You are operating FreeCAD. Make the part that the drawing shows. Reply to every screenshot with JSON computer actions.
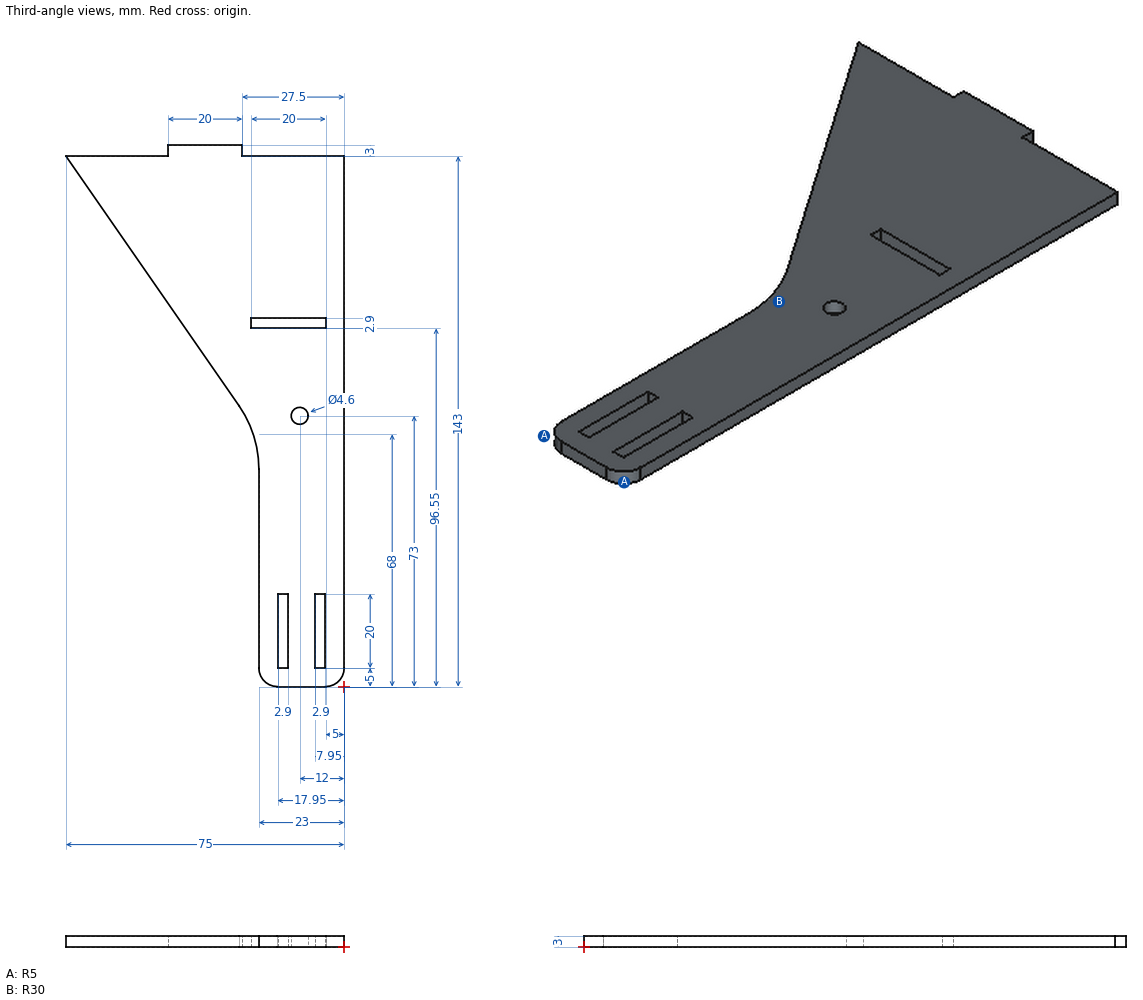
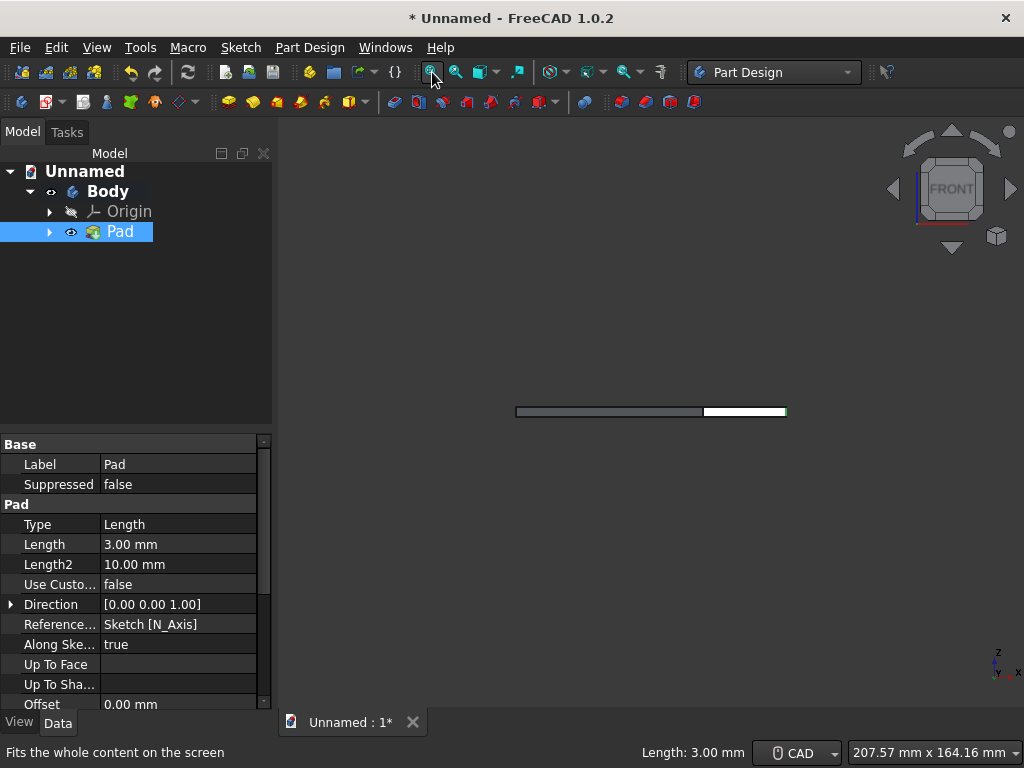
{"action": "left_click", "coordinate": [432, 72]}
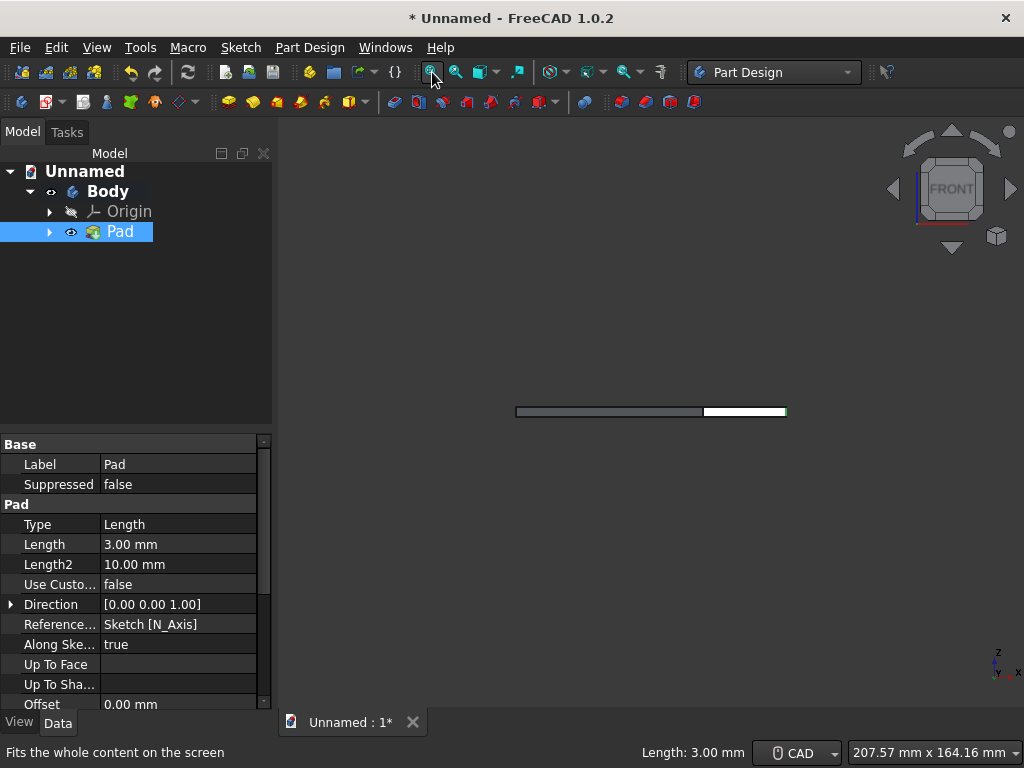
{"action": "scroll", "coordinate": [703, 411], "scroll_direction": "up", "scroll_amount": 7}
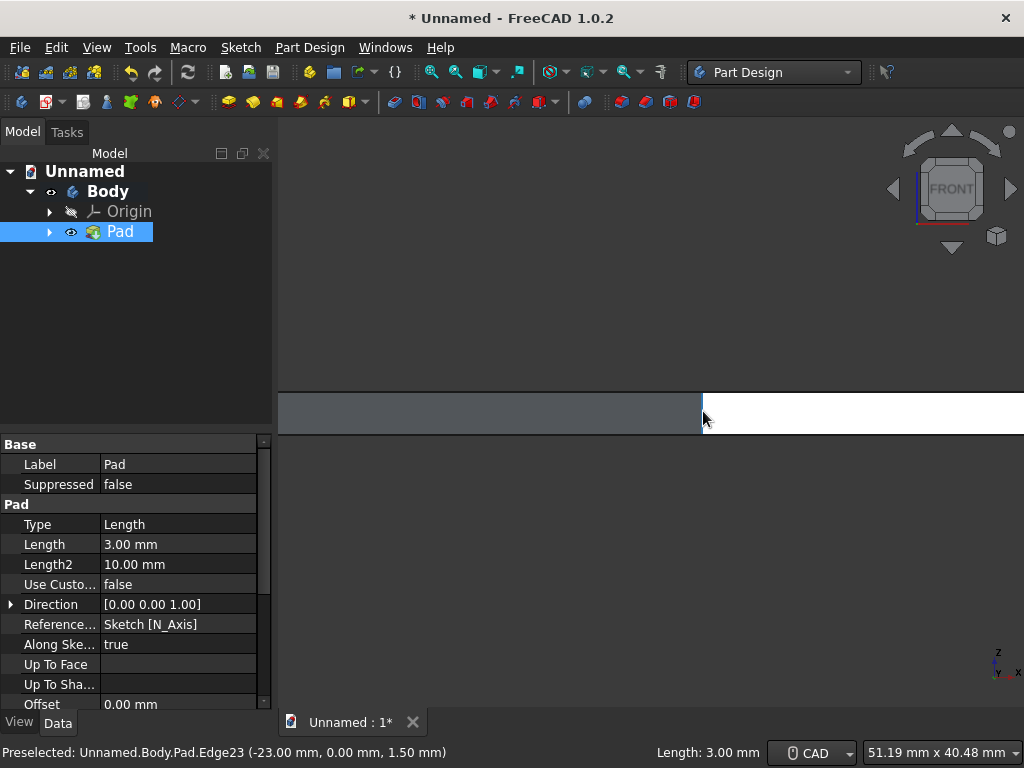
{"action": "left_click", "coordinate": [702, 413], "text": "ctrl"}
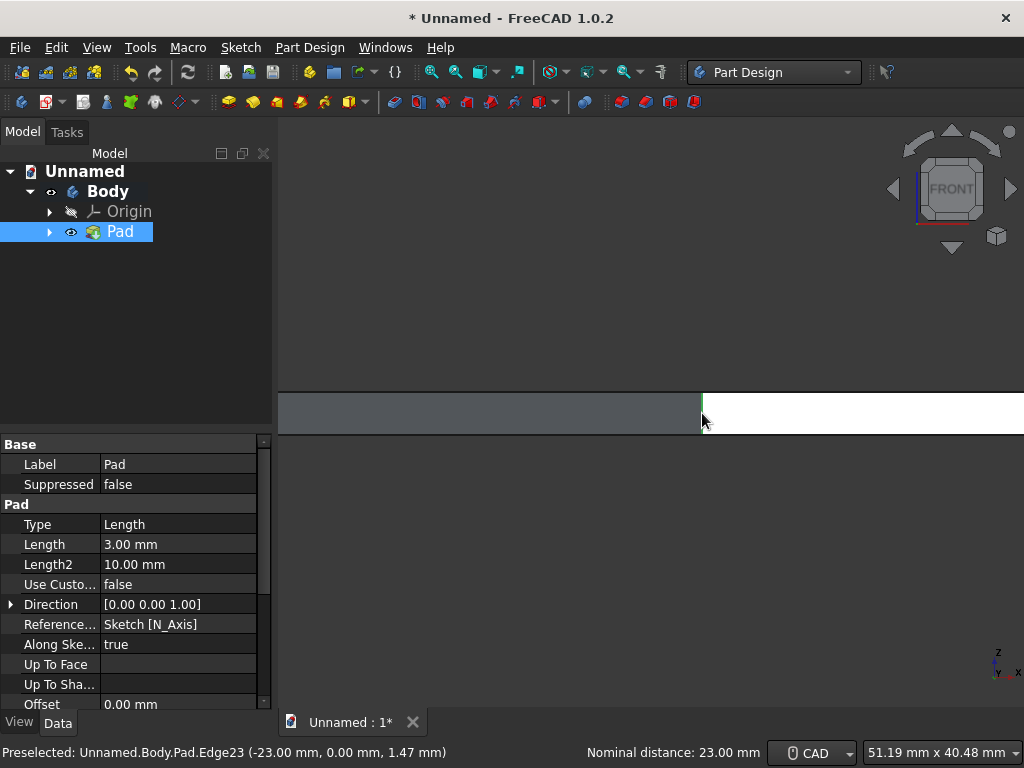
{"action": "left_click", "coordinate": [622, 102]}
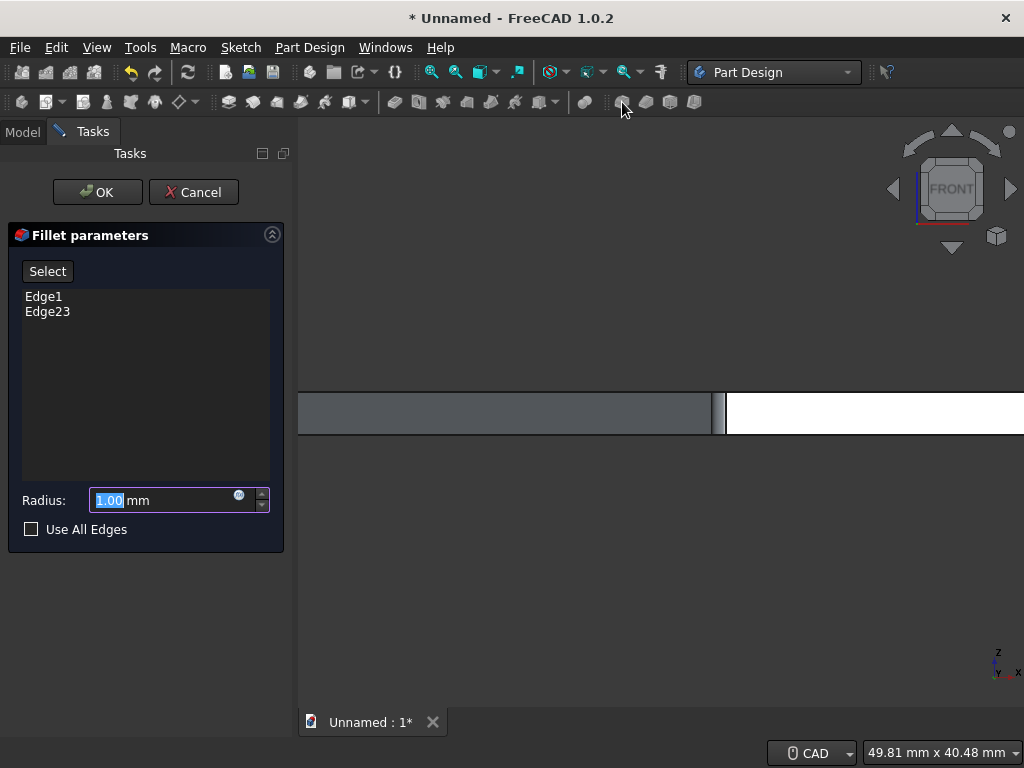
{"action": "type", "text": "5"}
{"action": "key", "text": "Tab"}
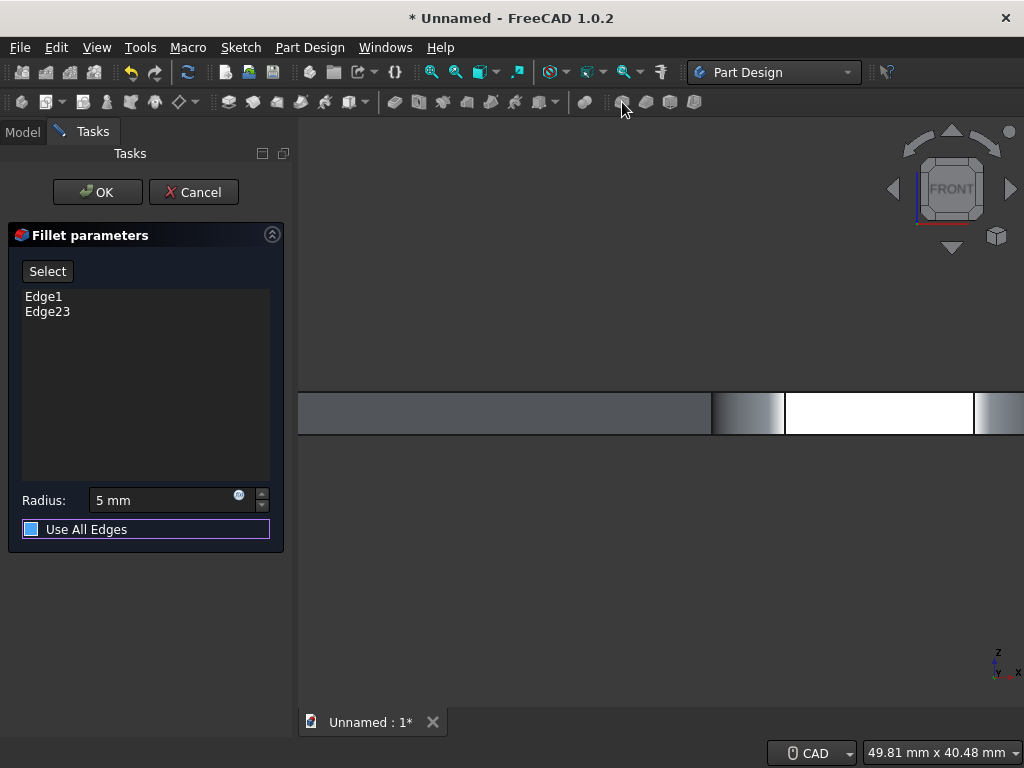
{"action": "left_click", "coordinate": [98, 192]}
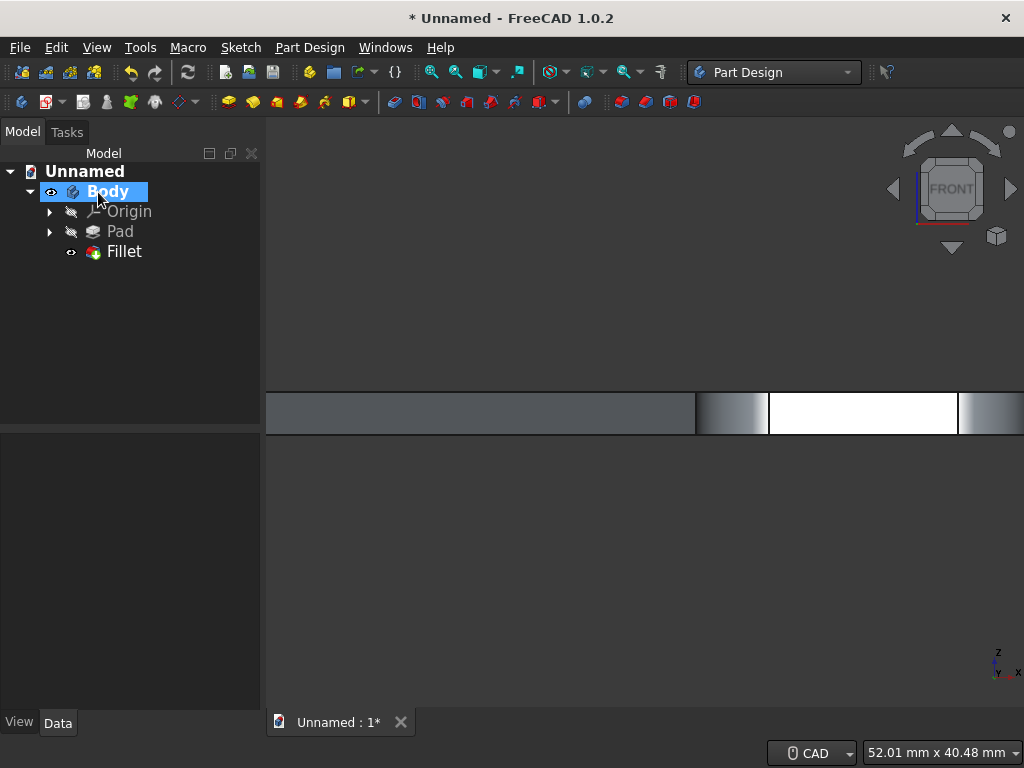
{"action": "key", "text": "v f"}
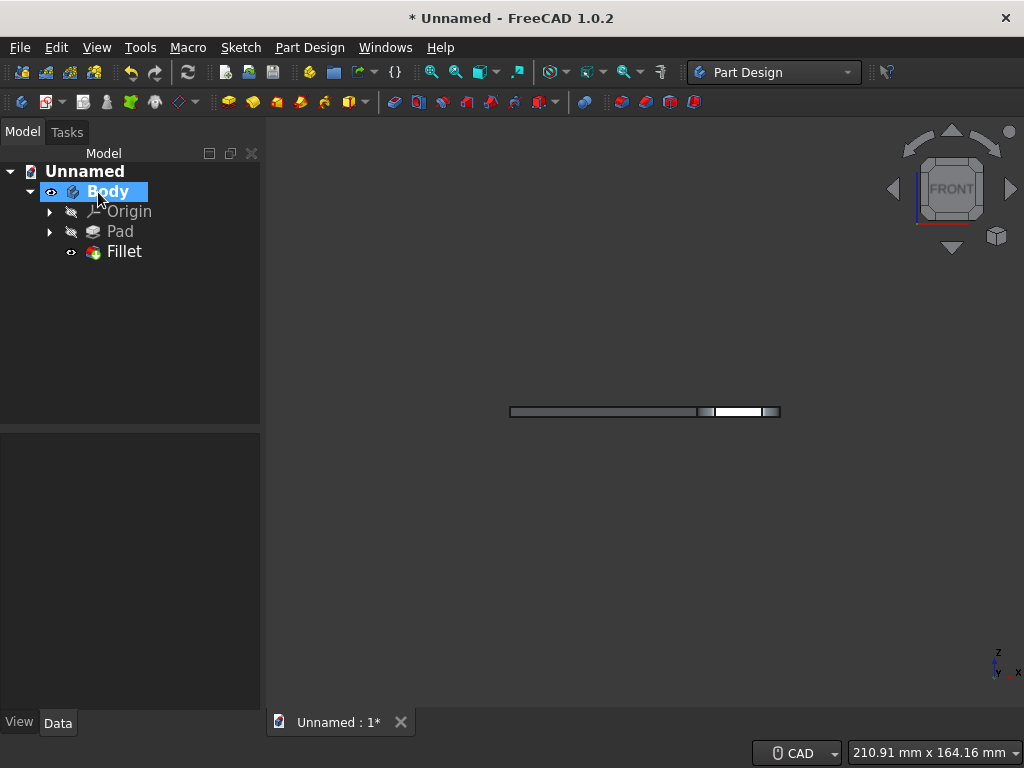
{"action": "scroll", "coordinate": [697, 411], "scroll_direction": "up", "scroll_amount": 7}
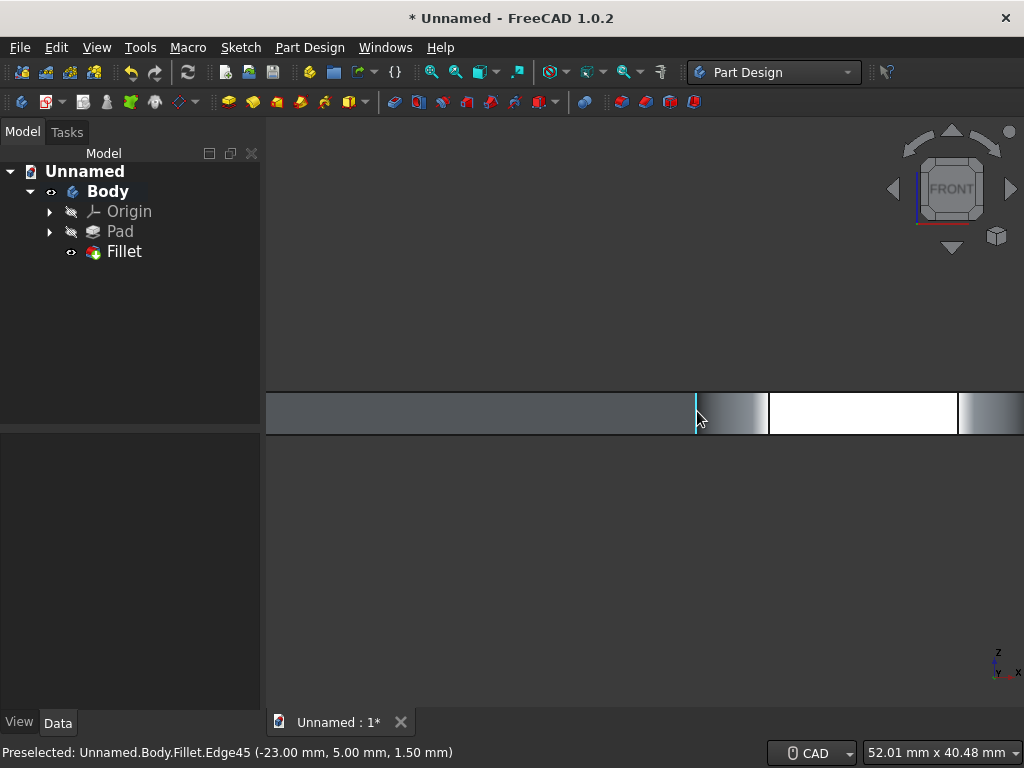
{"action": "key", "text": "v f"}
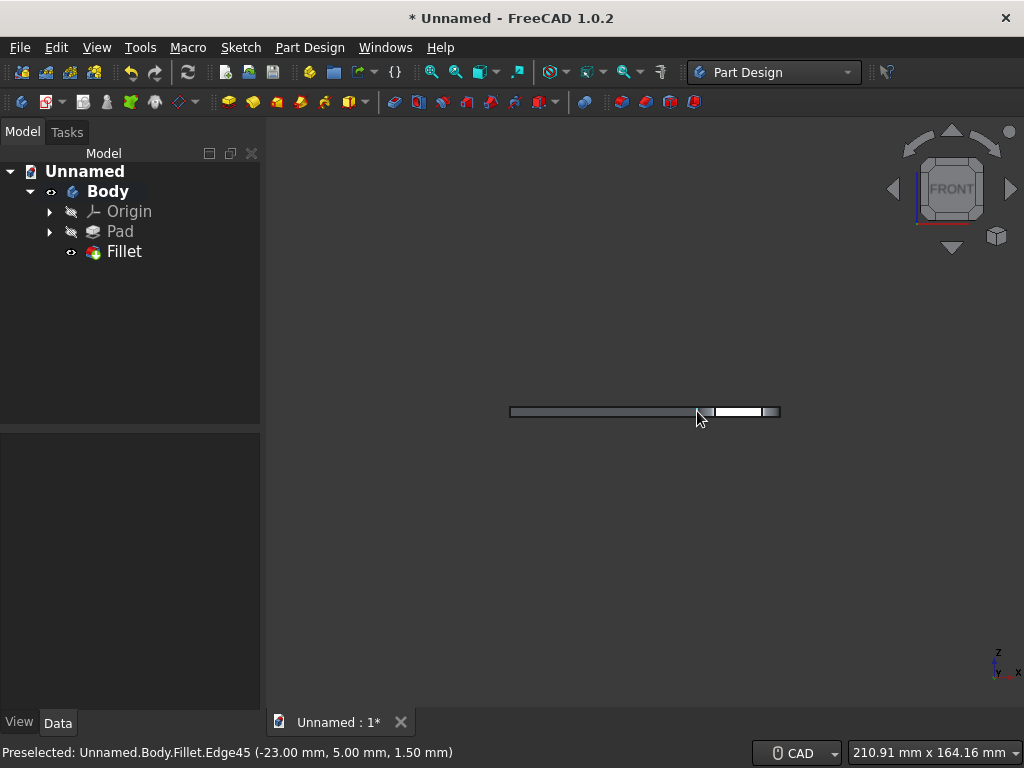
{"action": "key", "text": "0"}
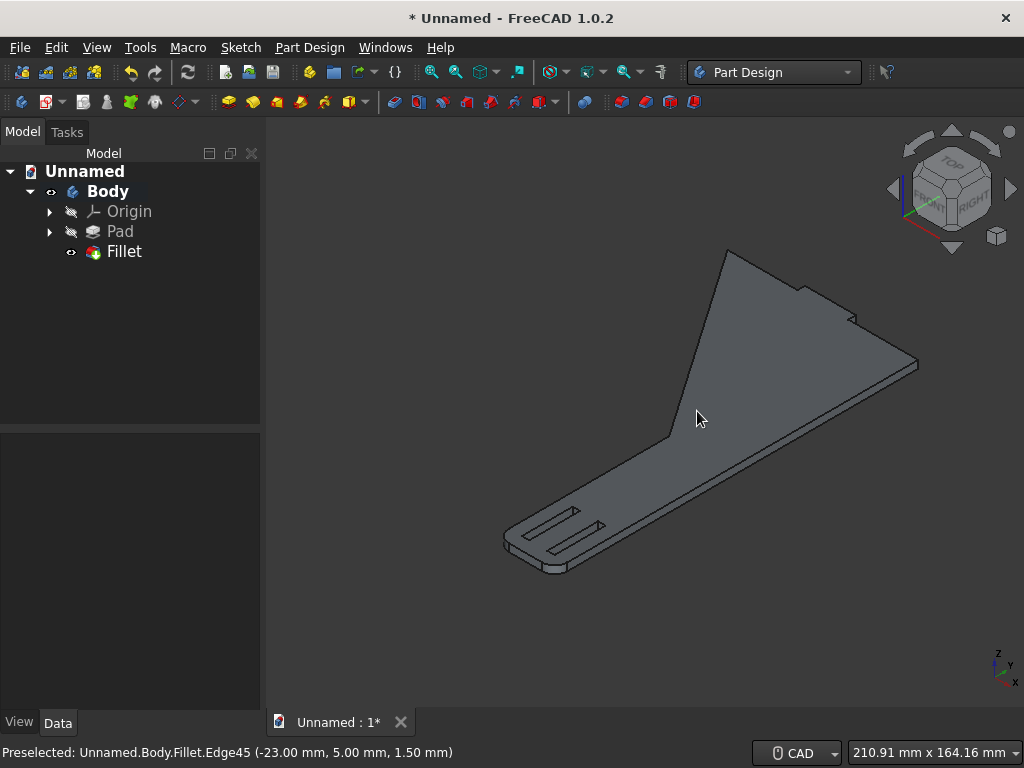
{"action": "scroll", "coordinate": [669, 440], "scroll_direction": "up", "scroll_amount": 7}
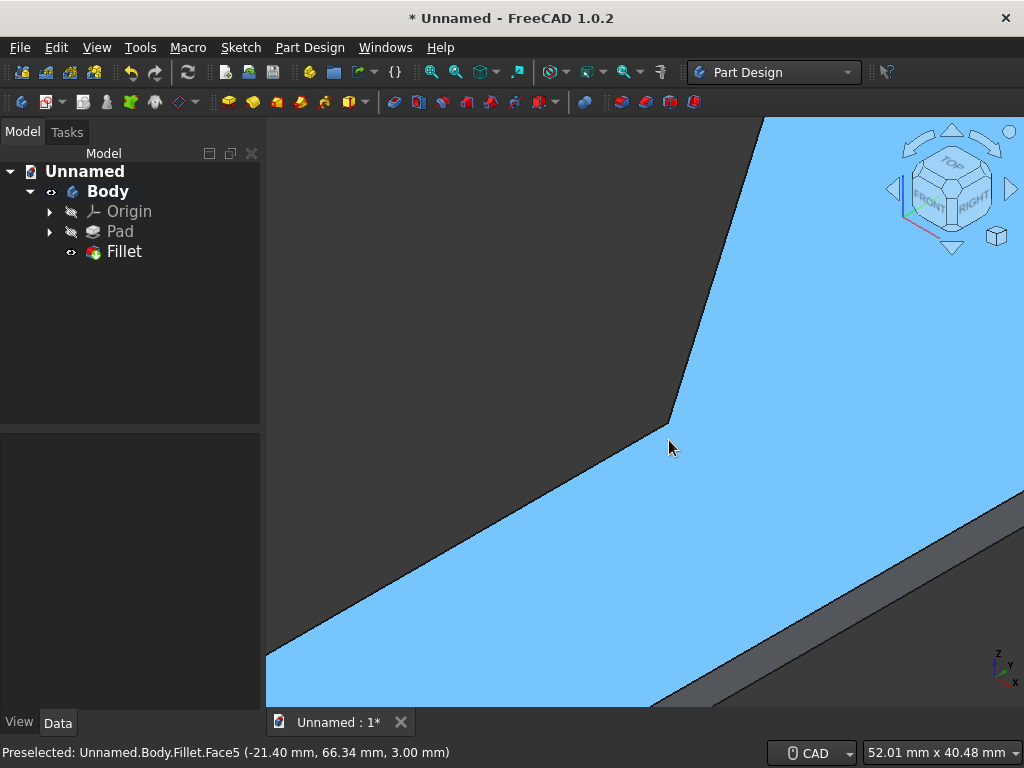
{"action": "left_click", "coordinate": [432, 72]}